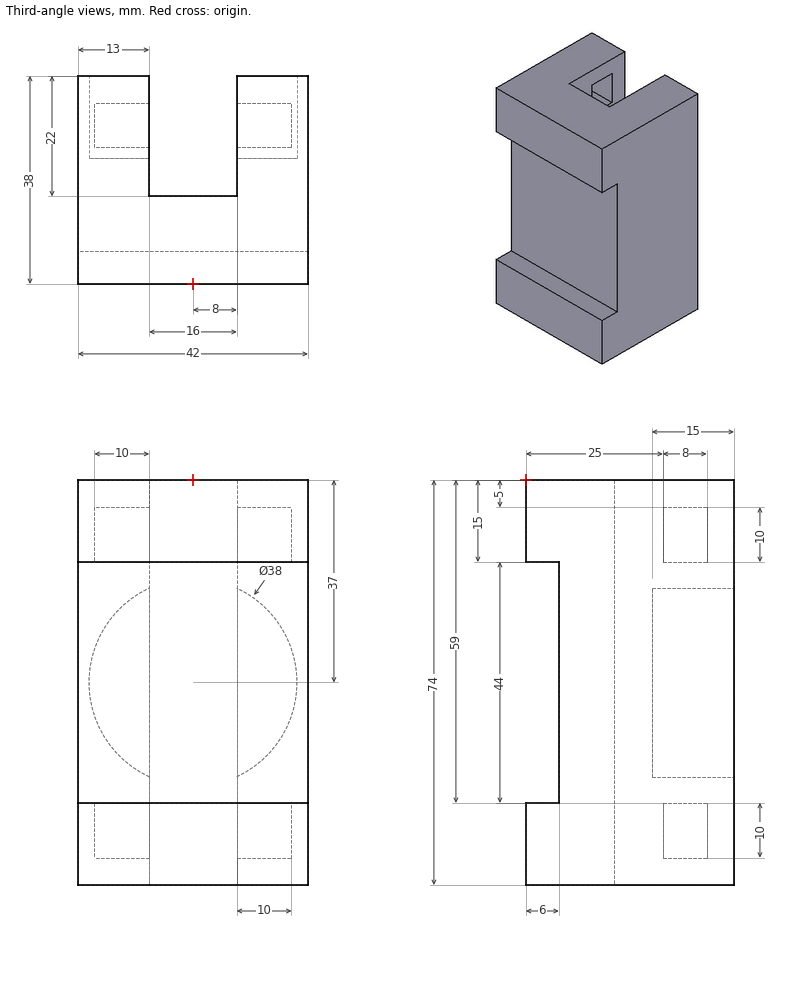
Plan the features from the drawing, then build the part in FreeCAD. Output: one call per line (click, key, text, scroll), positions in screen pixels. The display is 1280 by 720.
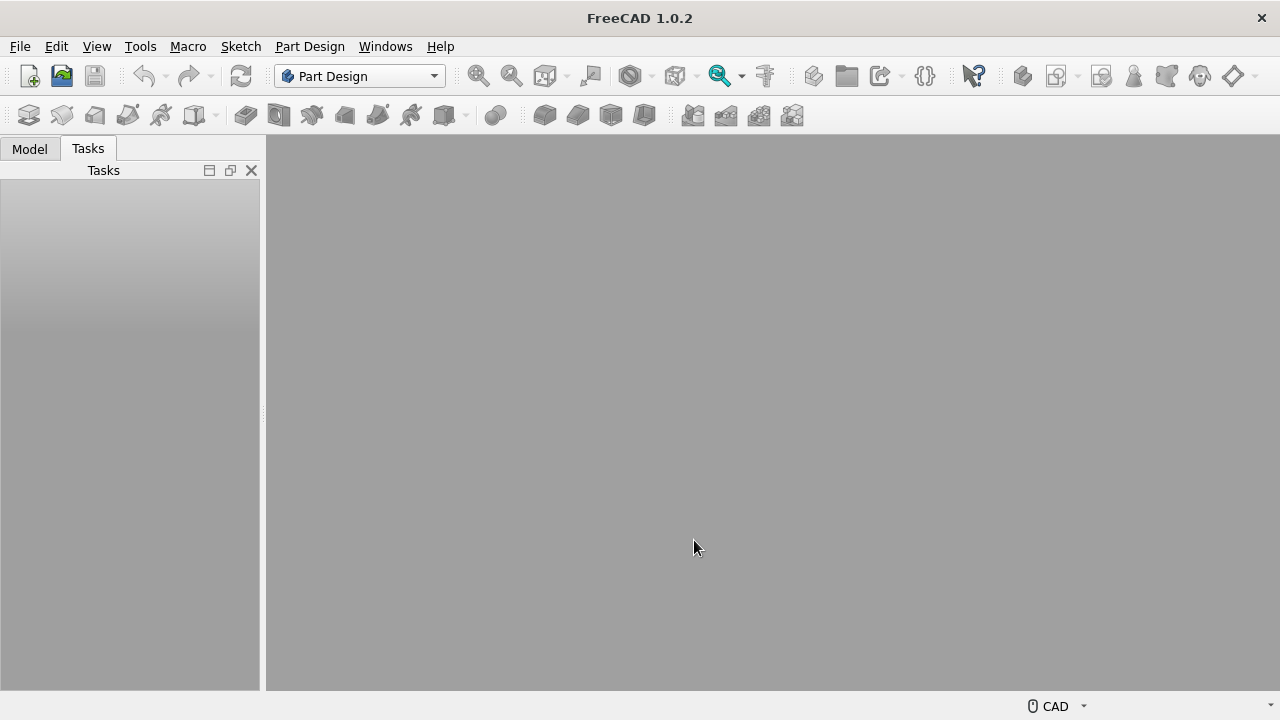
key(ctrl+n)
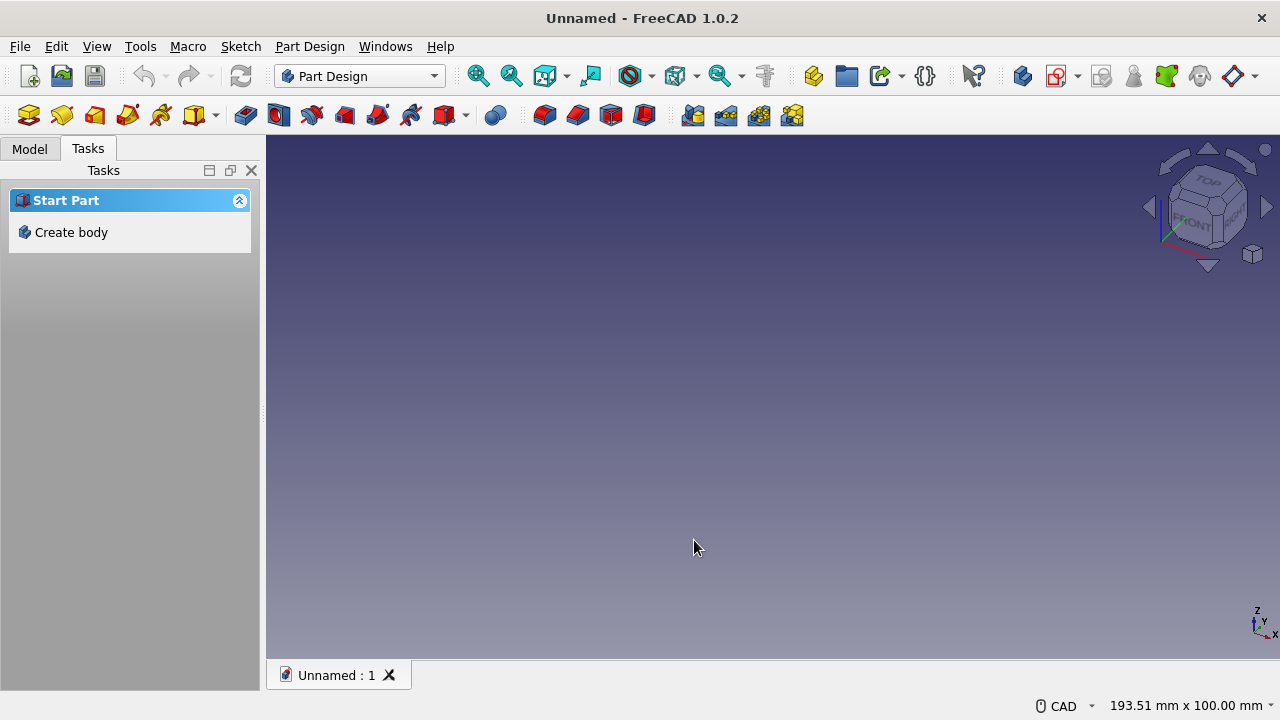
click(1056, 76)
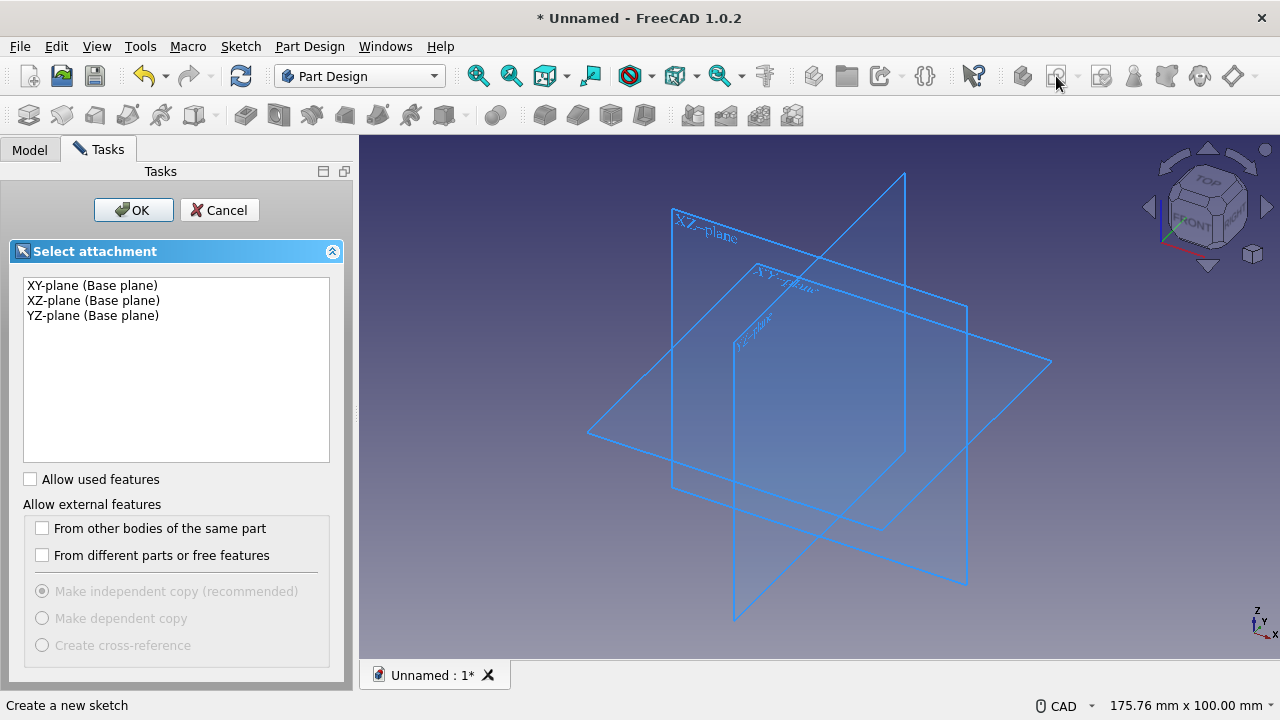
click(84, 286)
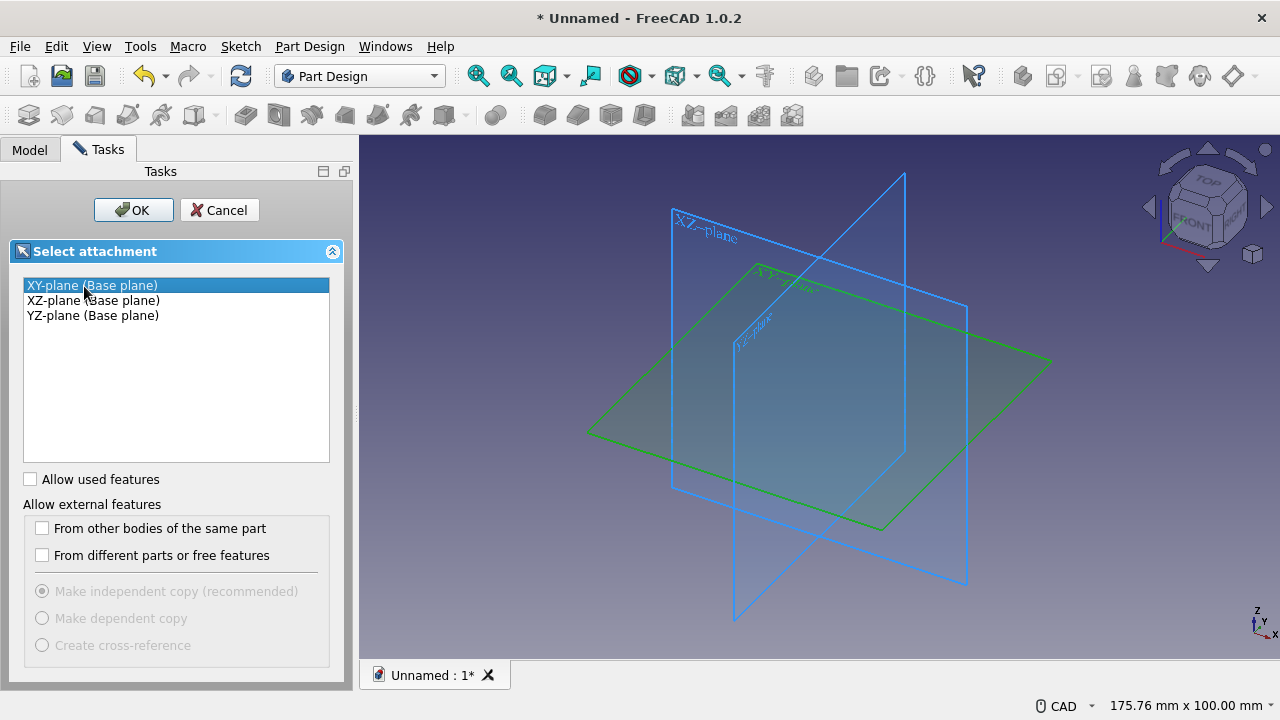
click(134, 210)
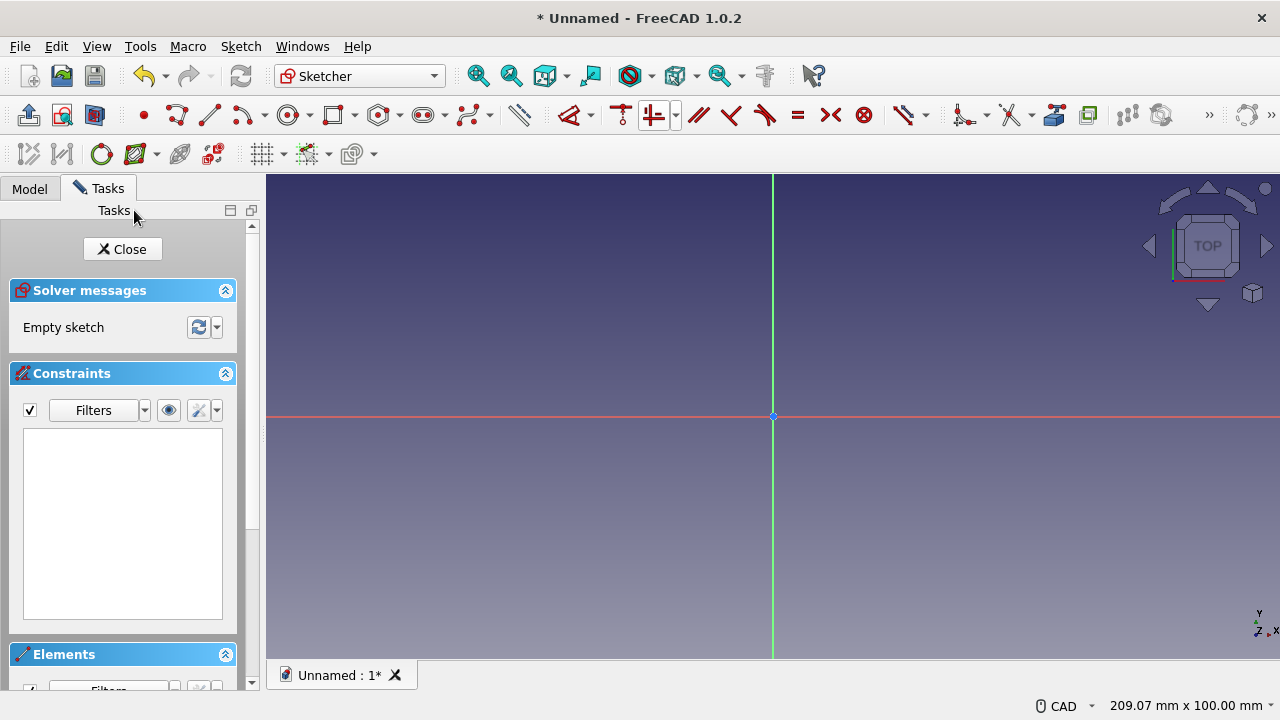
scroll(912, 202, up, 2)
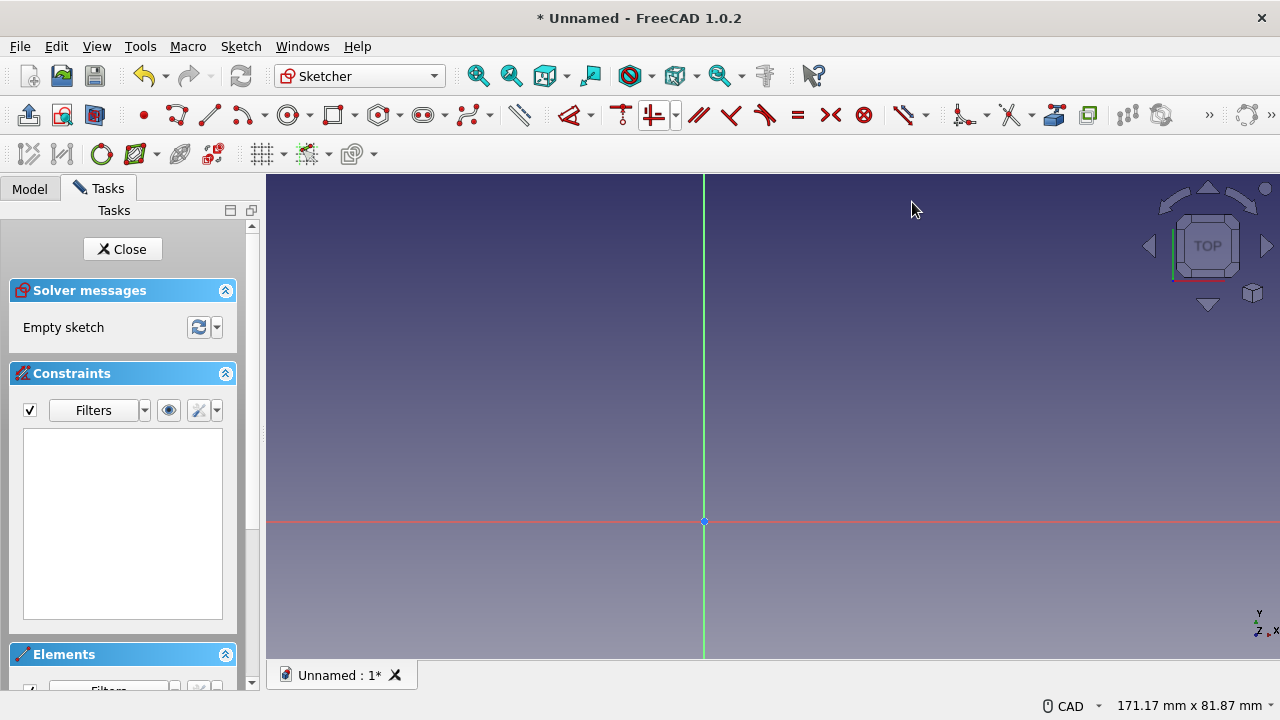
key(g)
key(m)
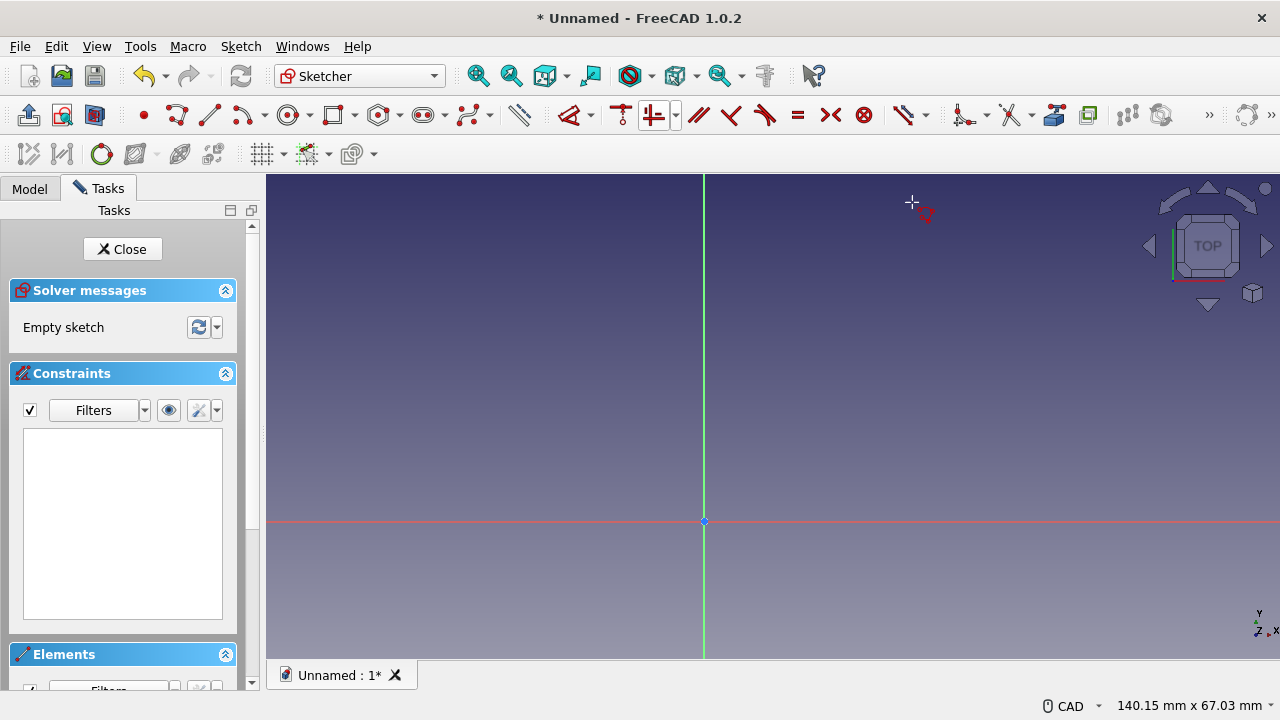
click(762, 406)
click(646, 406)
click(646, 247)
click(552, 247)
click(552, 522)
click(856, 513)
click(856, 247)
click(762, 247)
click(762, 407)
key(Escape)
key(Escape)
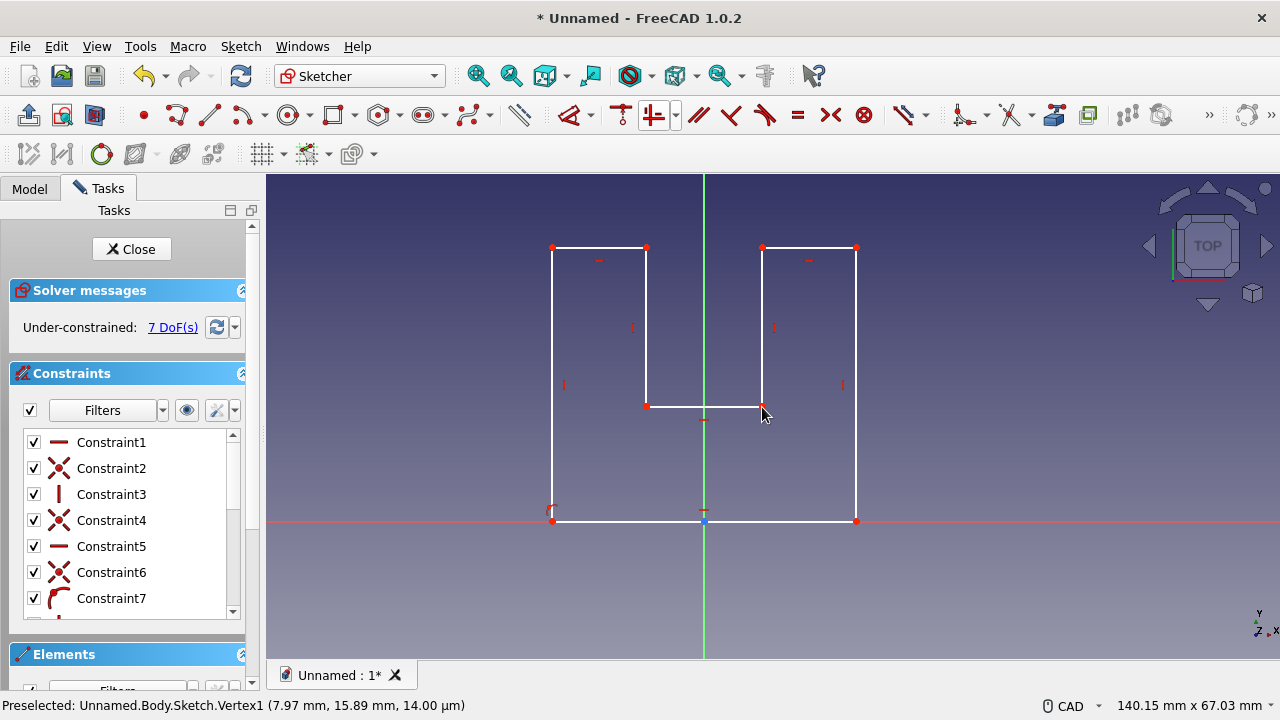
click(727, 407)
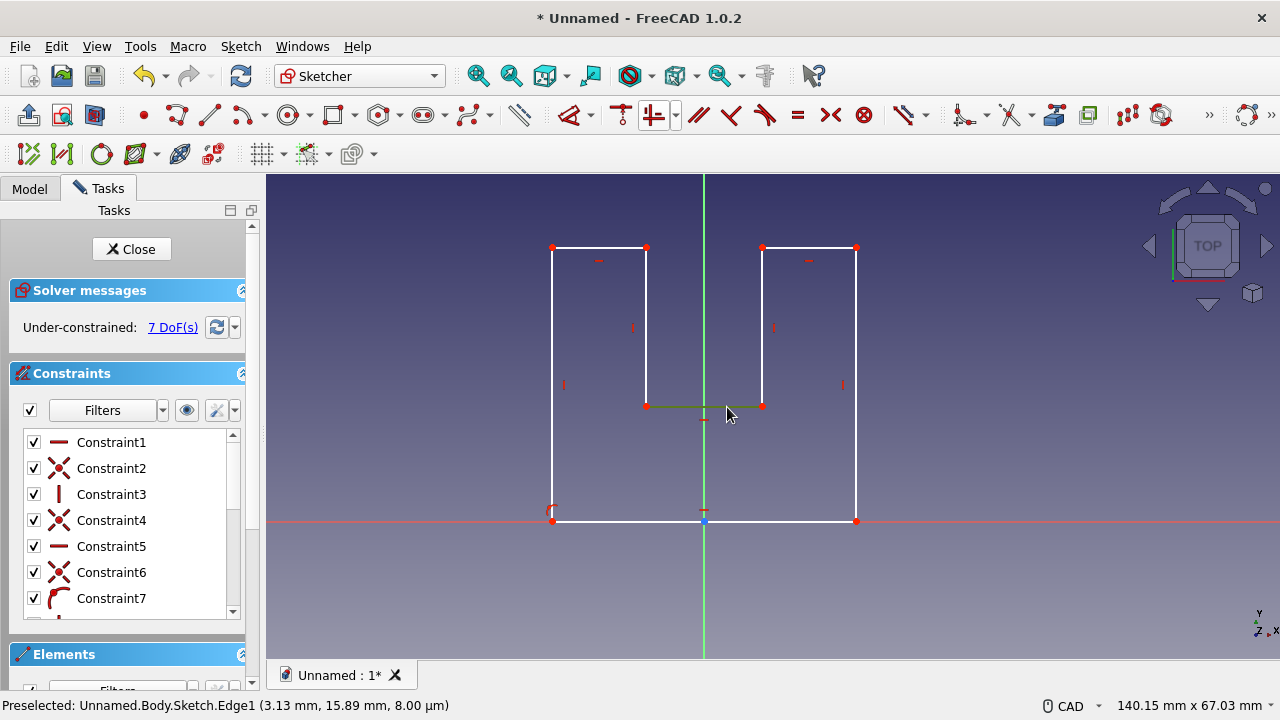
key(l)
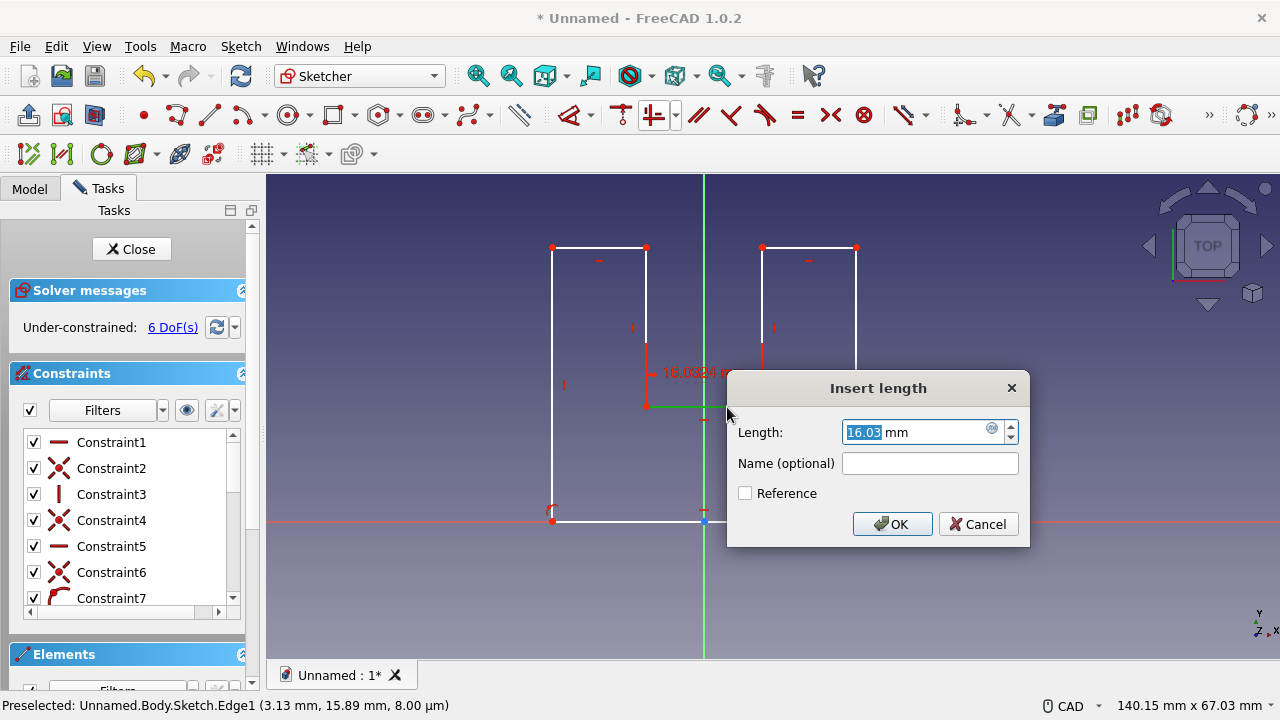
text(16)
key(Return)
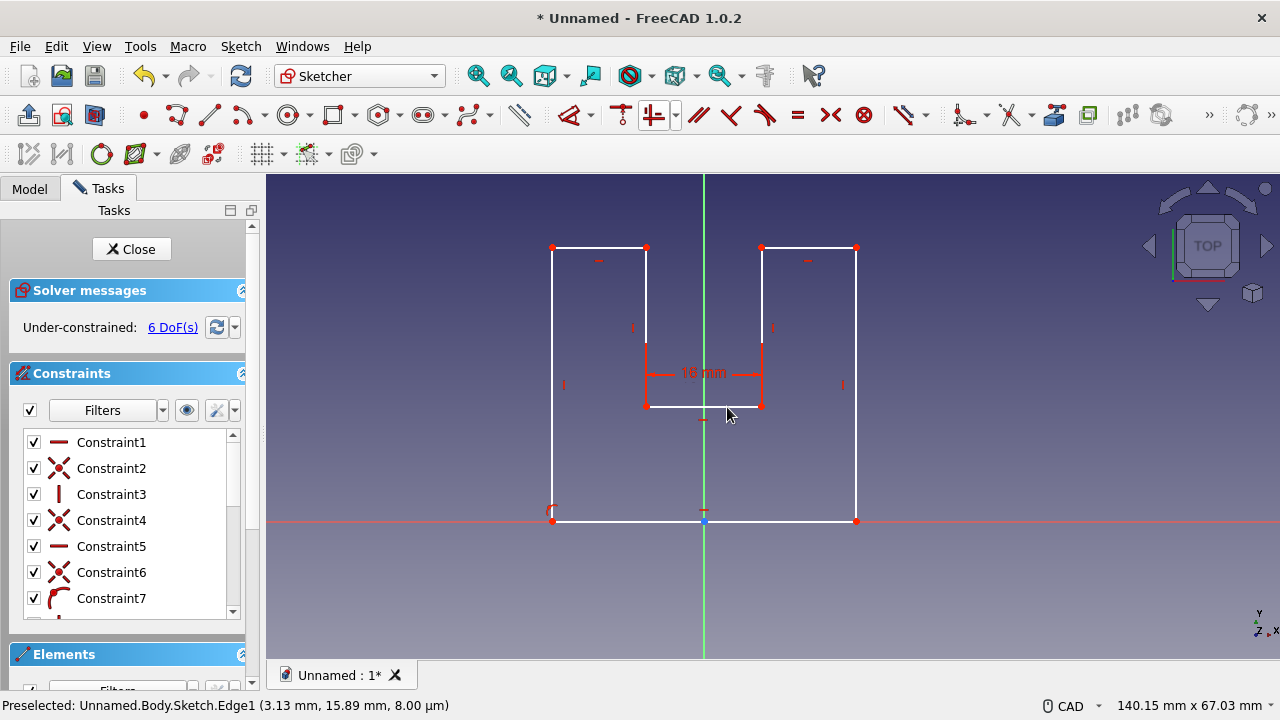
click(646, 359)